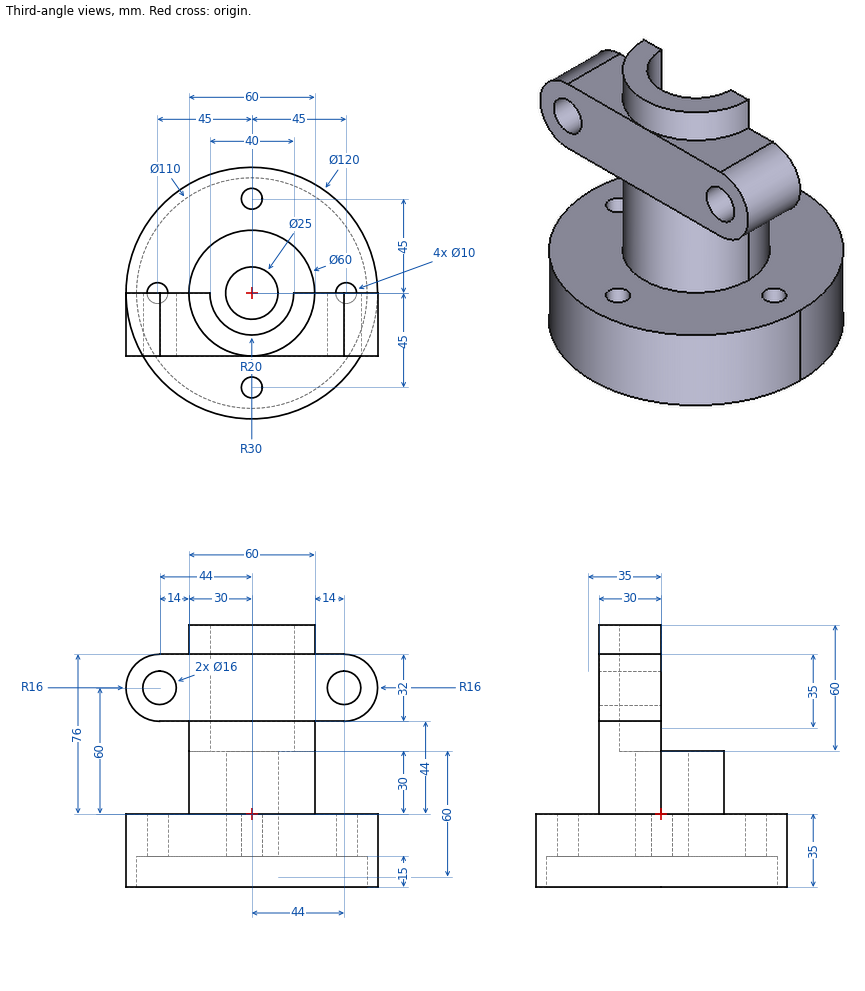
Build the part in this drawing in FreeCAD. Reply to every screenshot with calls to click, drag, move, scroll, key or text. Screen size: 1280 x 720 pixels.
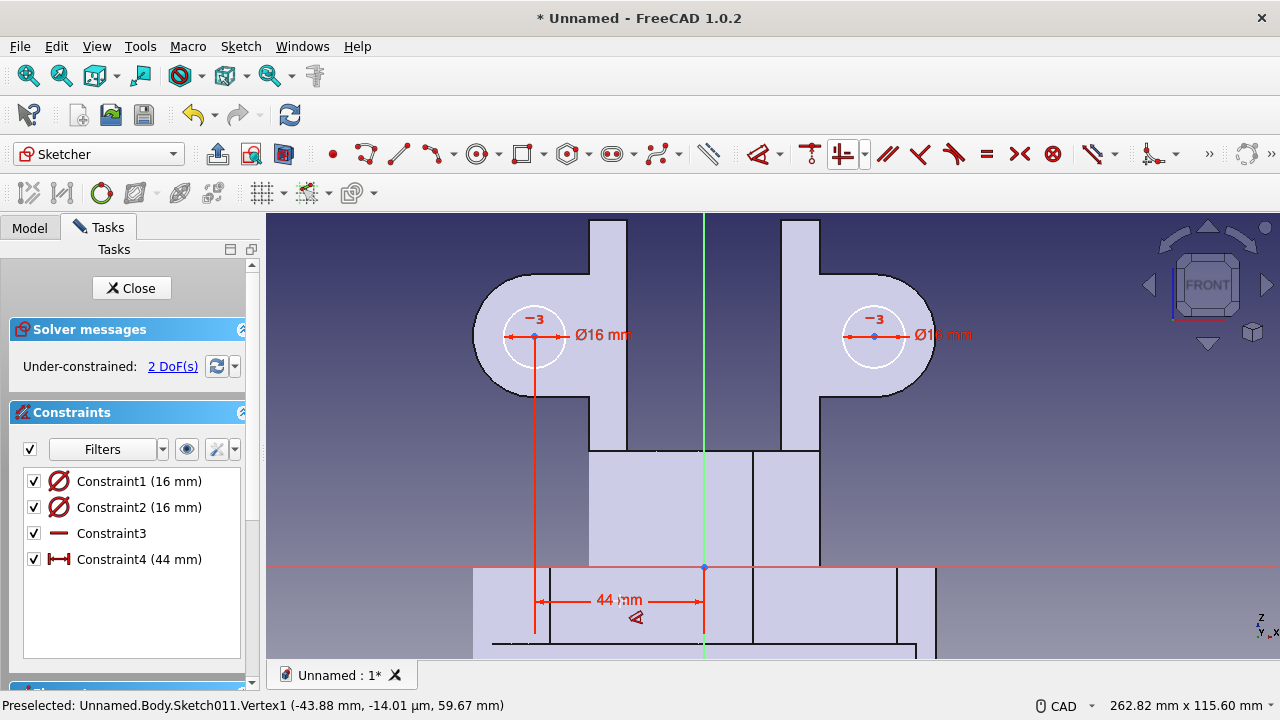
click(535, 337)
click(501, 452)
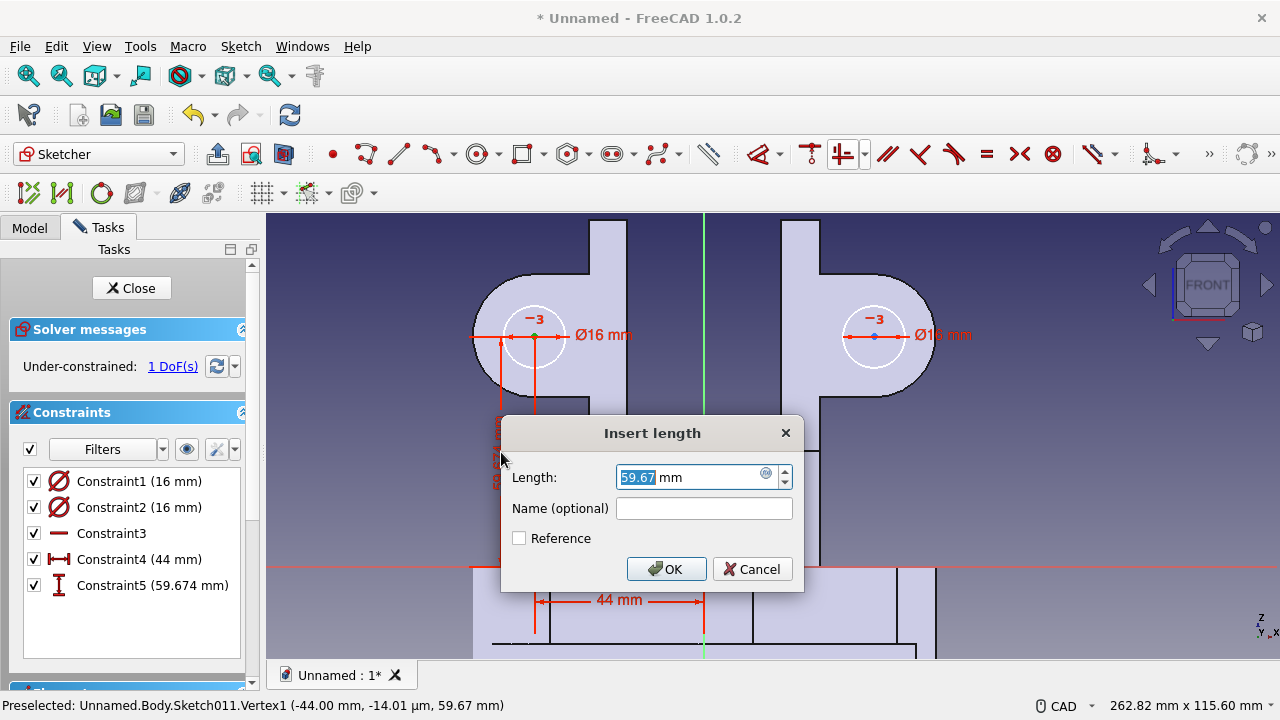
text(60)
key(Return)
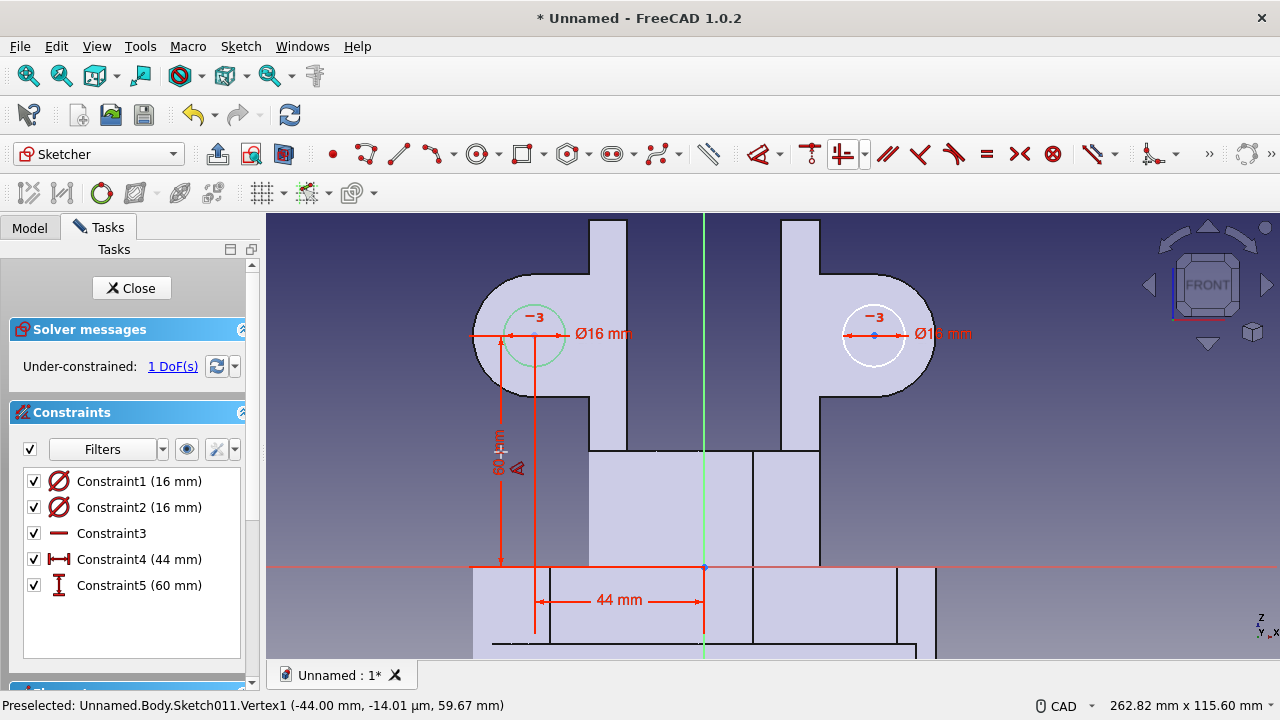
click(874, 336)
click(789, 601)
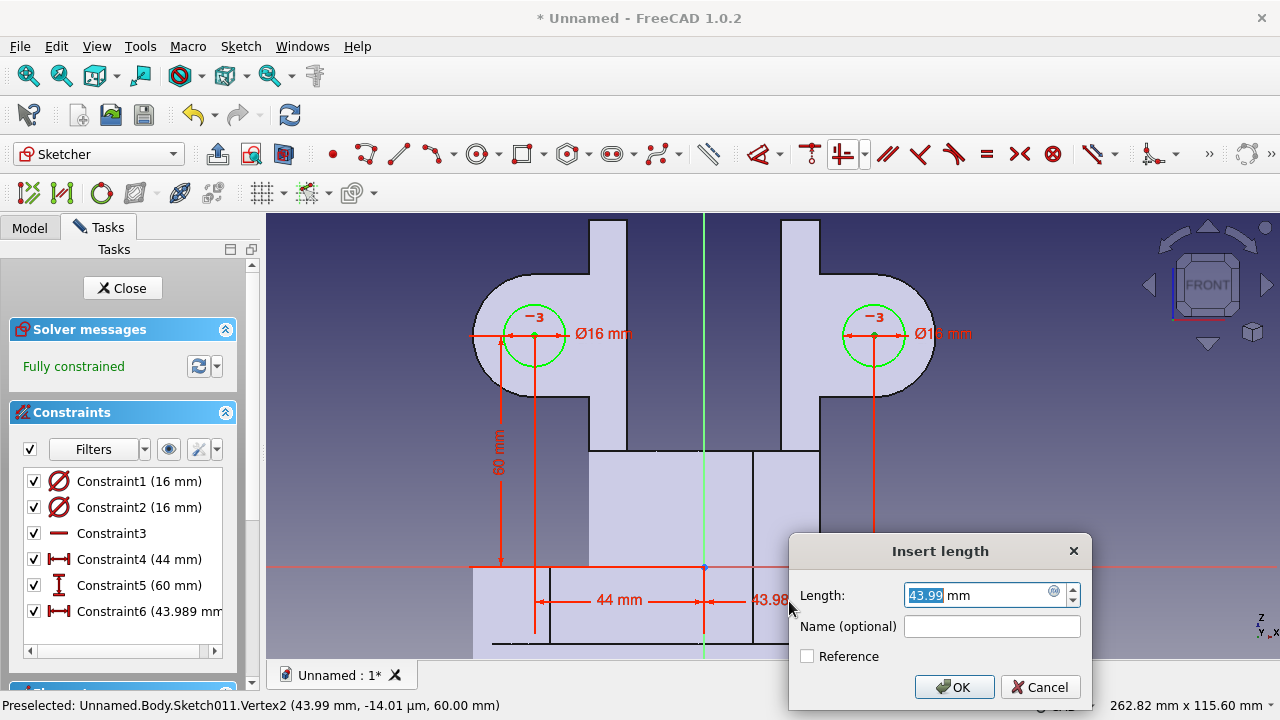
text(44)
key(Return)
key(Escape)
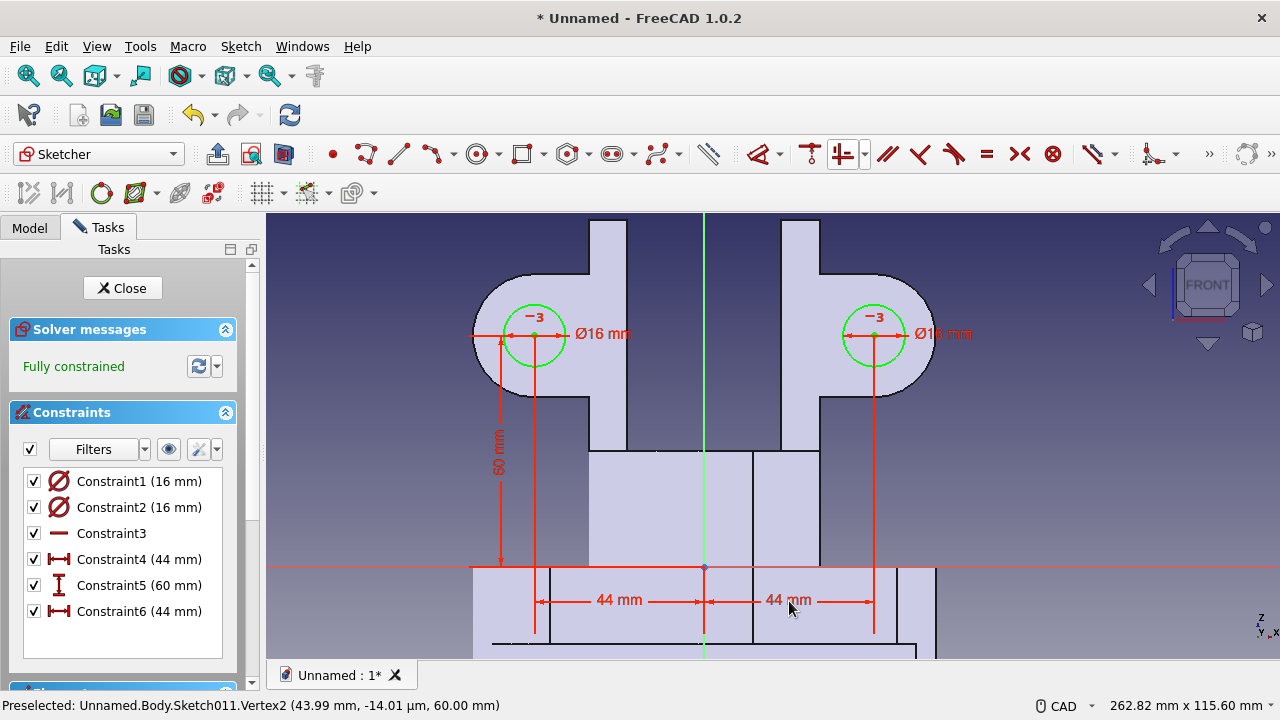
click(123, 288)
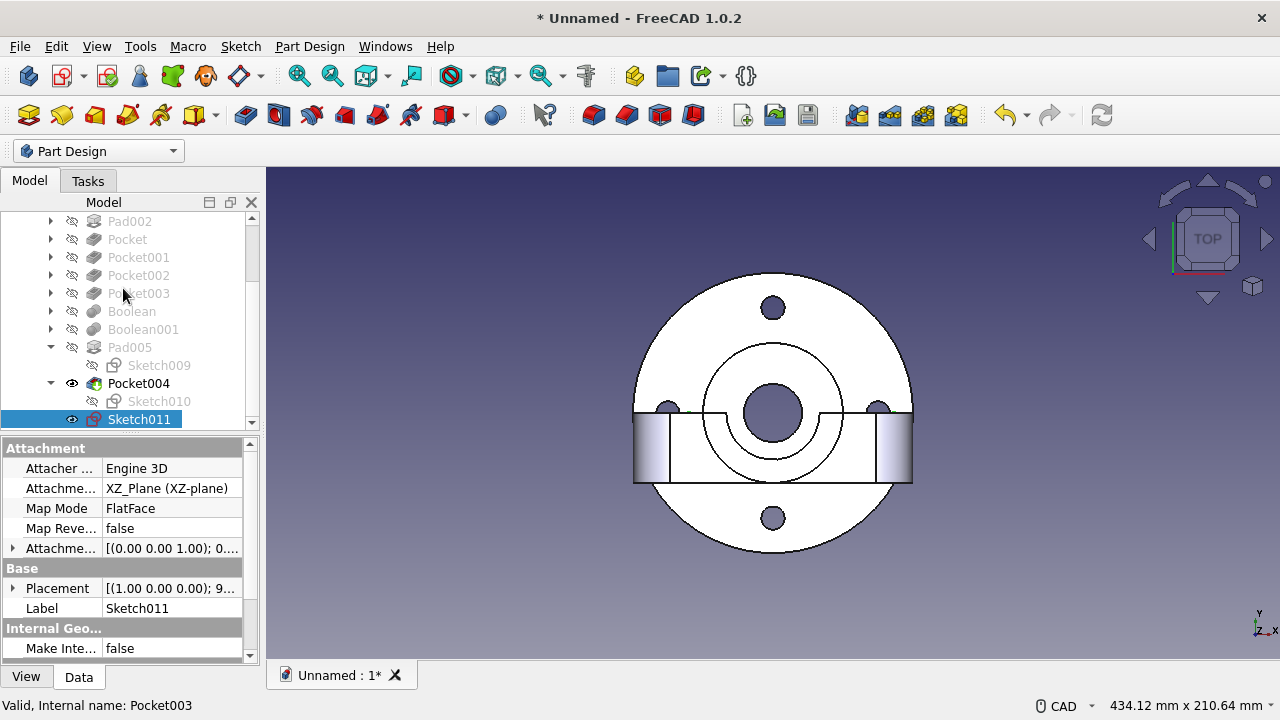
click(246, 116)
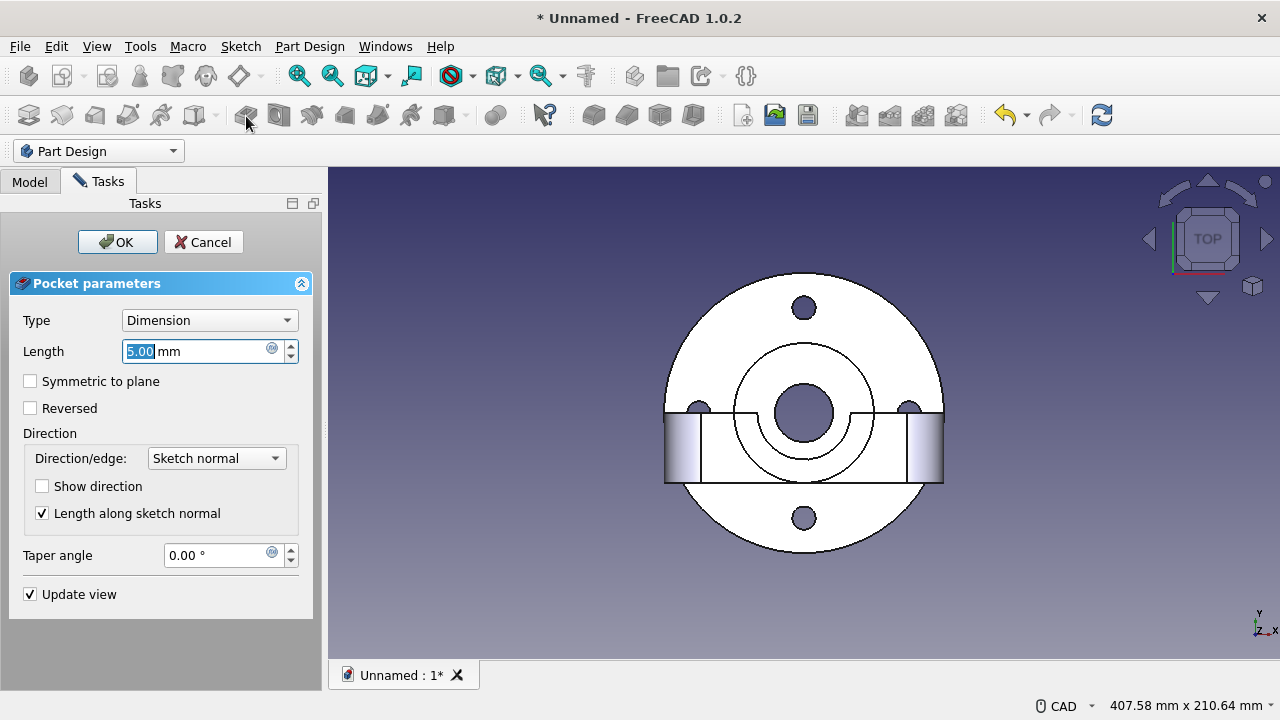
text(35)
key(Tab)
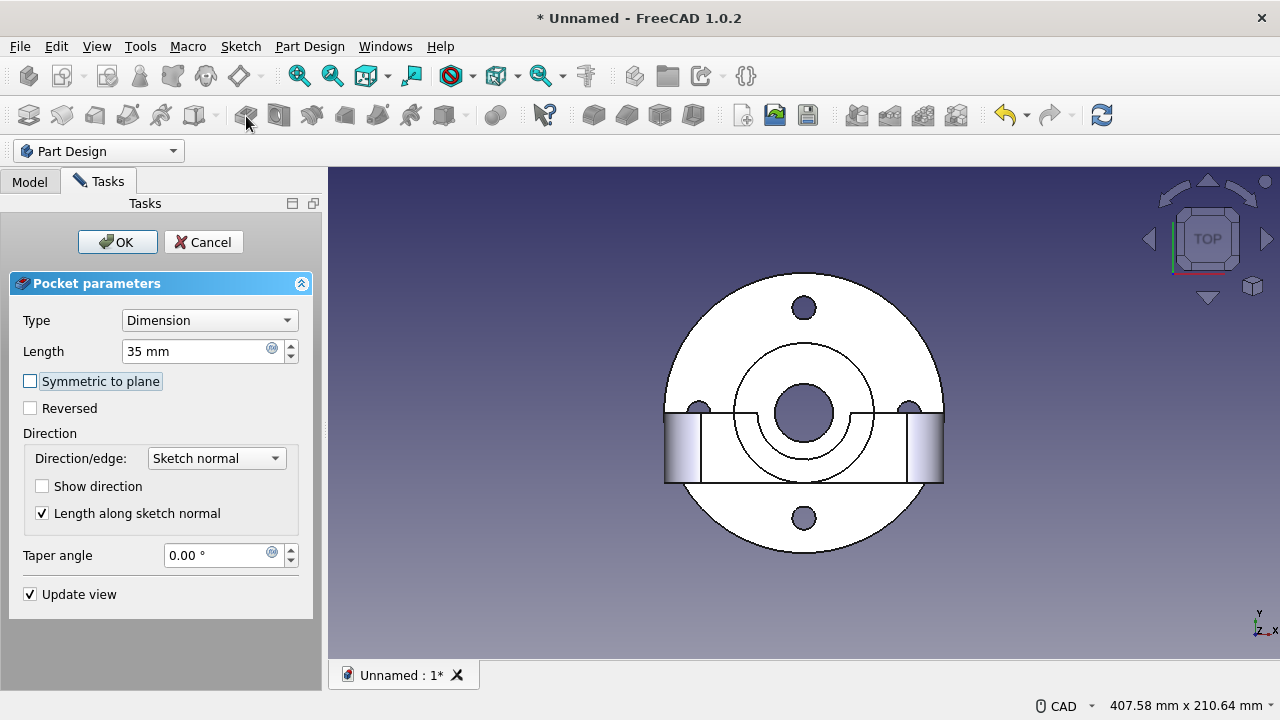
click(31, 408)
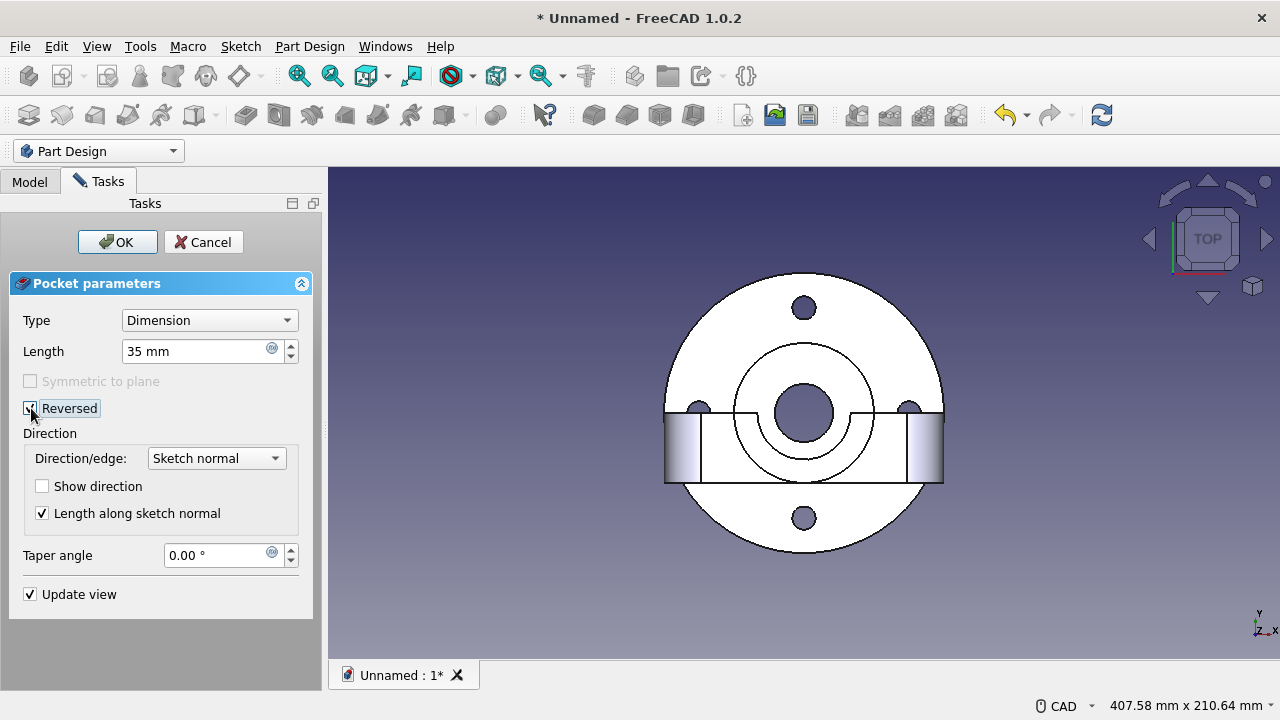
click(118, 242)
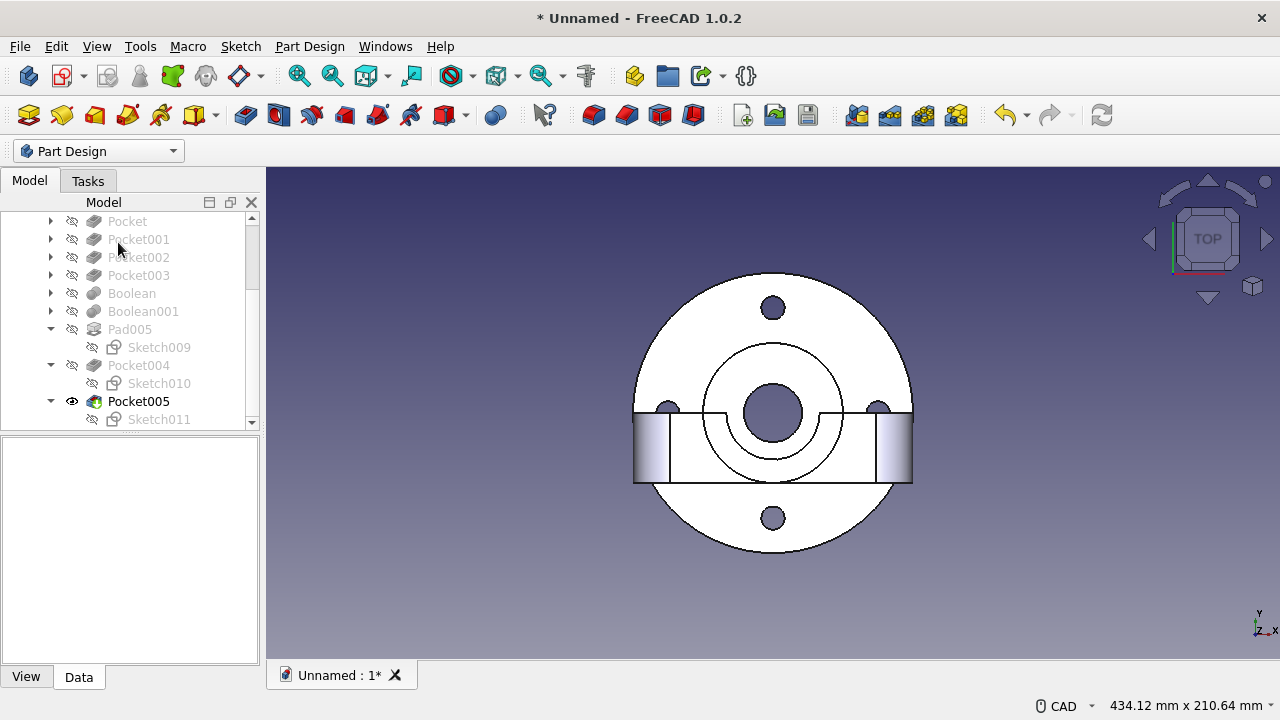
key(0)